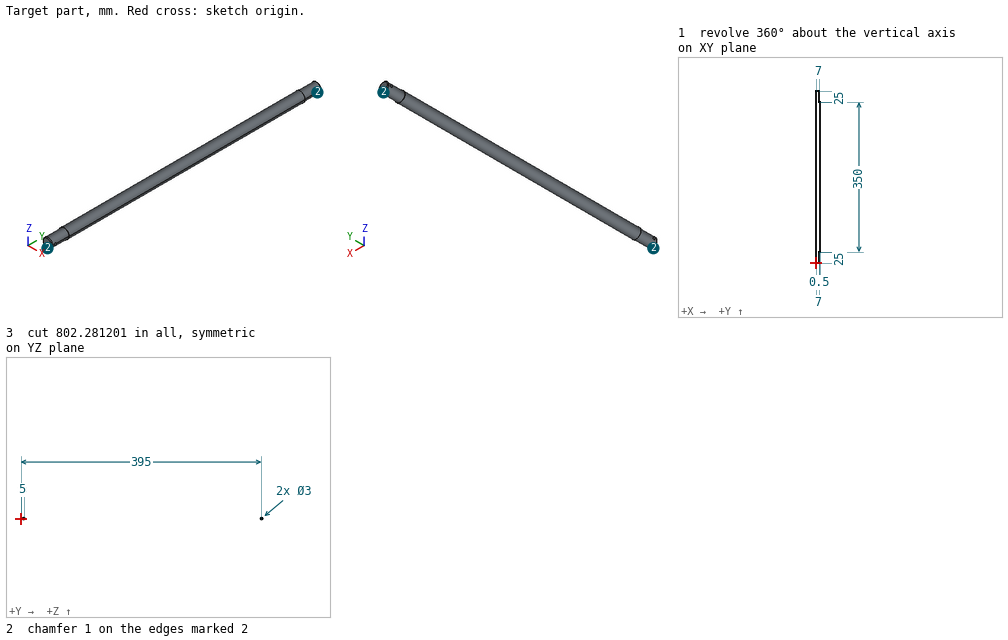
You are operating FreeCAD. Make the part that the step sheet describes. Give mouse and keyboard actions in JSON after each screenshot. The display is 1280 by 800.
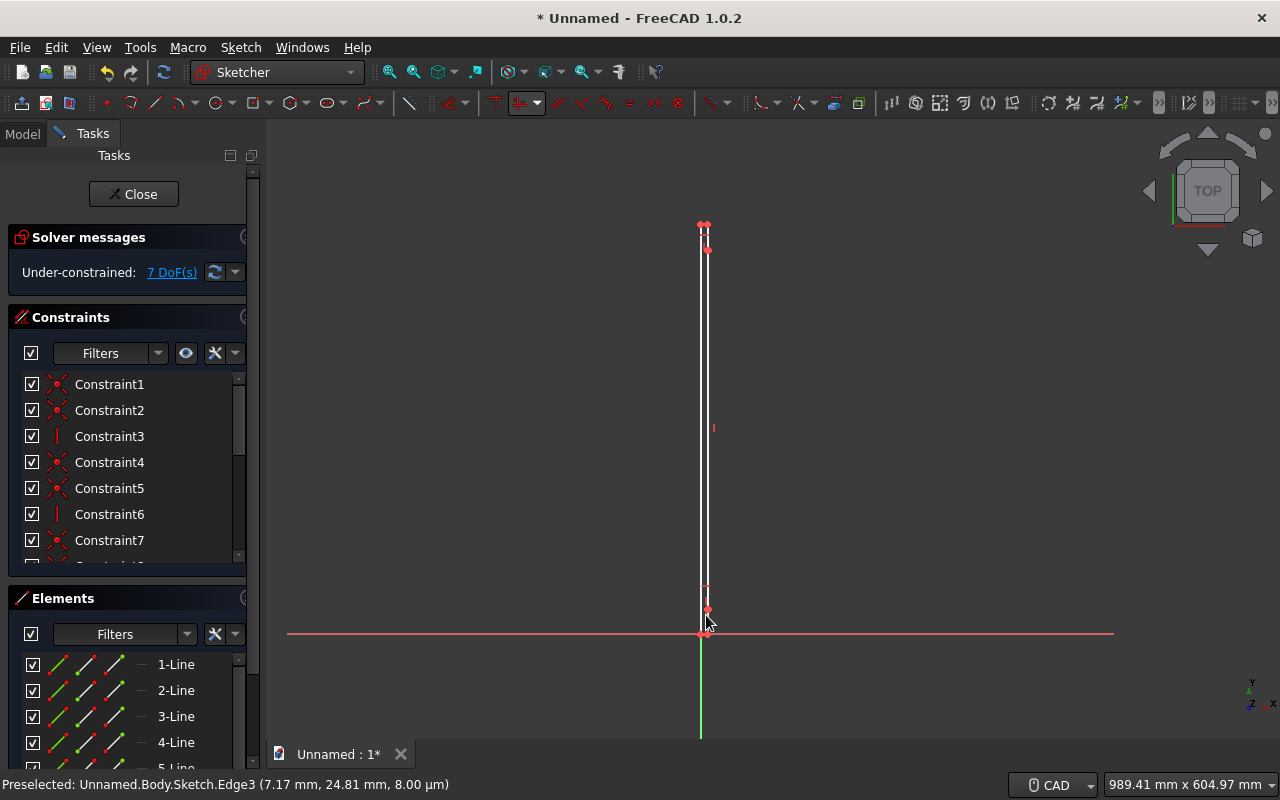
{"action": "scroll", "coordinate": [708, 250], "scroll_direction": "up", "scroll_amount": 14}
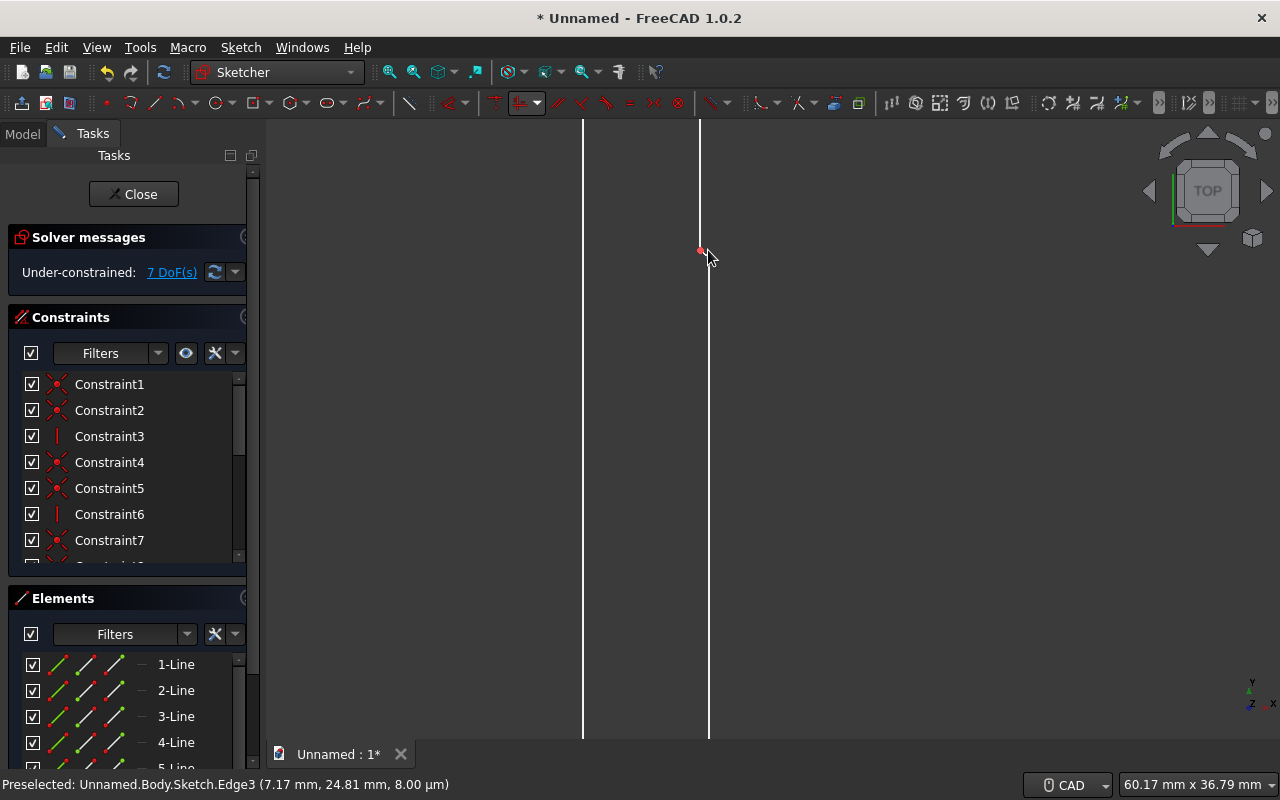
{"action": "scroll", "coordinate": [705, 254], "scroll_direction": "up", "scroll_amount": 4}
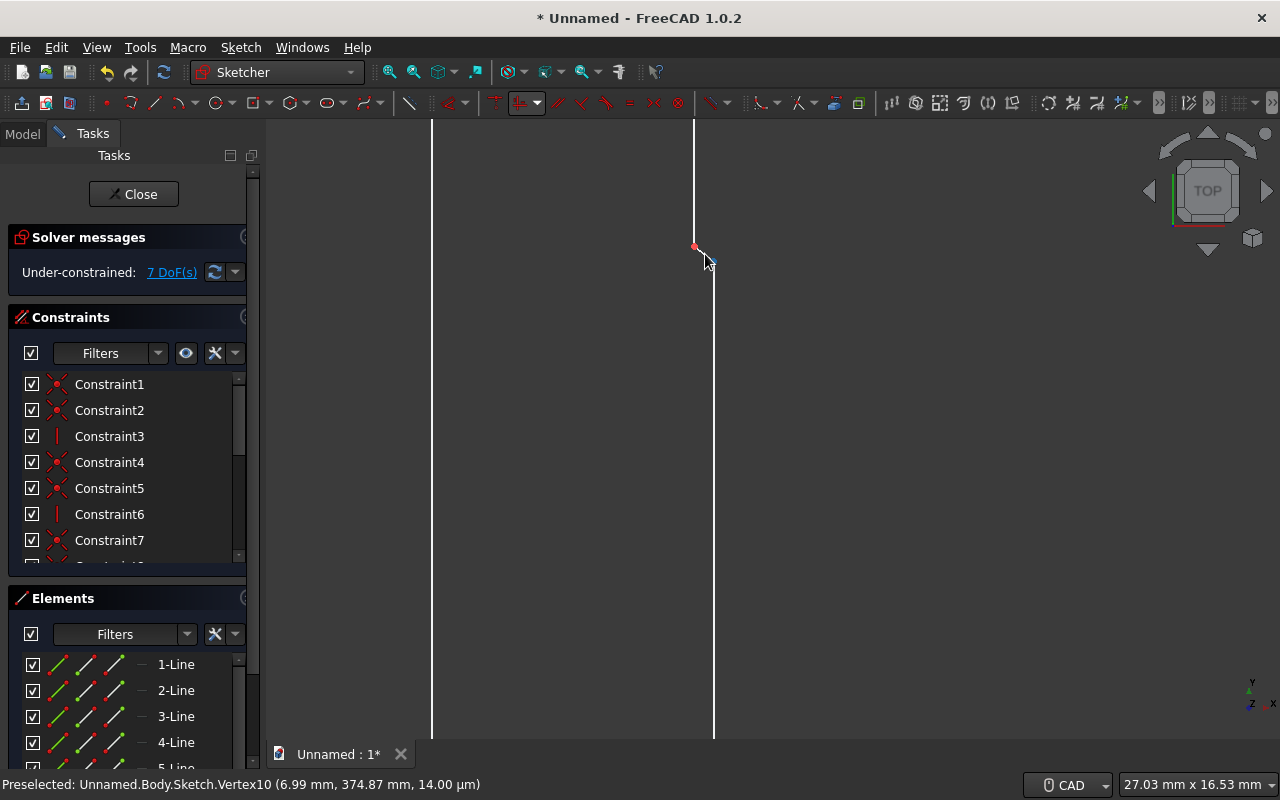
{"action": "left_click", "coordinate": [704, 254]}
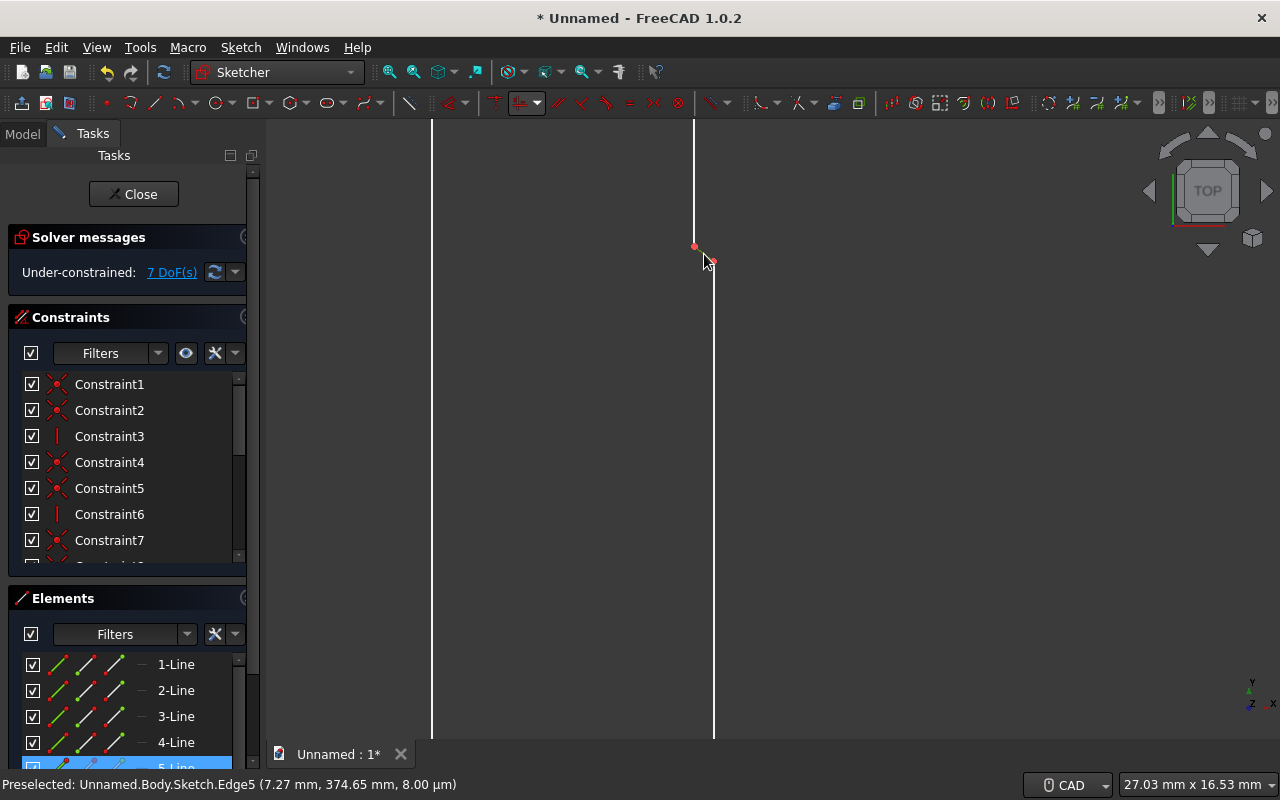
{"action": "key", "text": "h"}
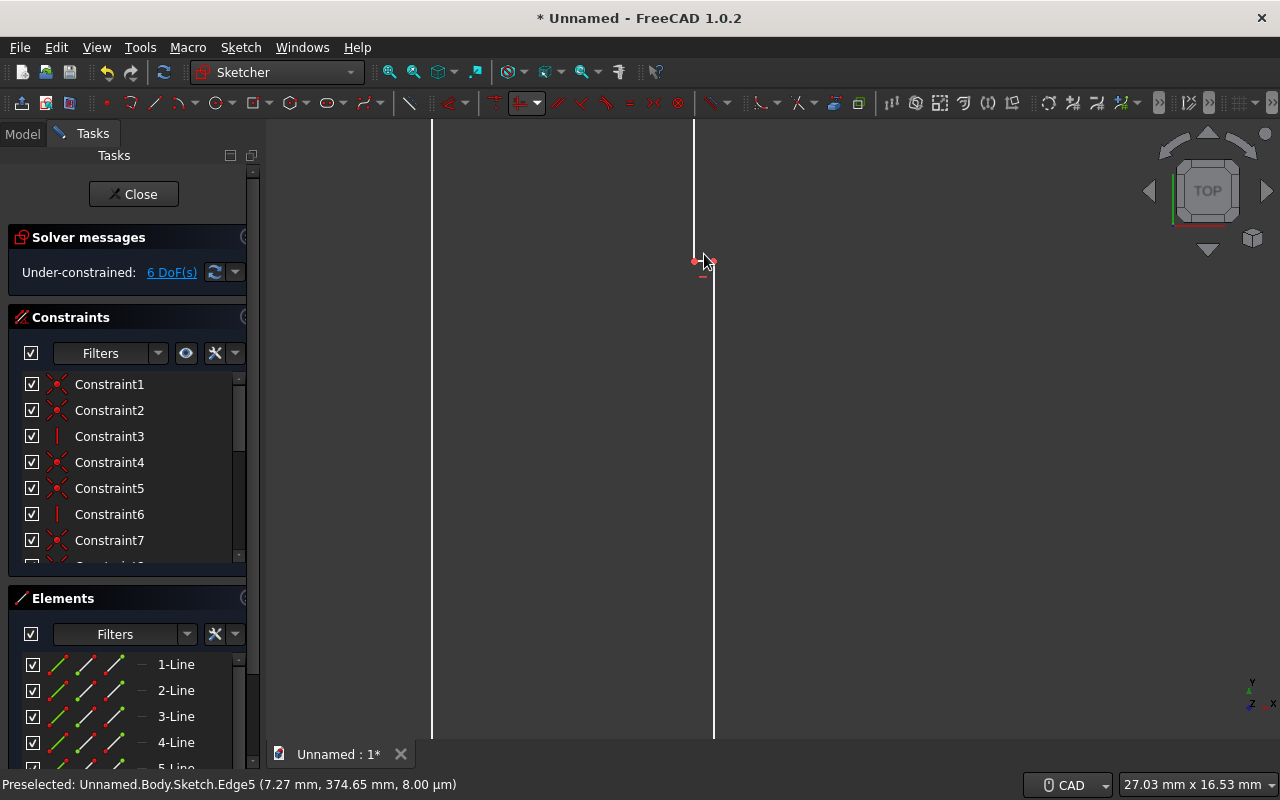
{"action": "left_click", "coordinate": [448, 104]}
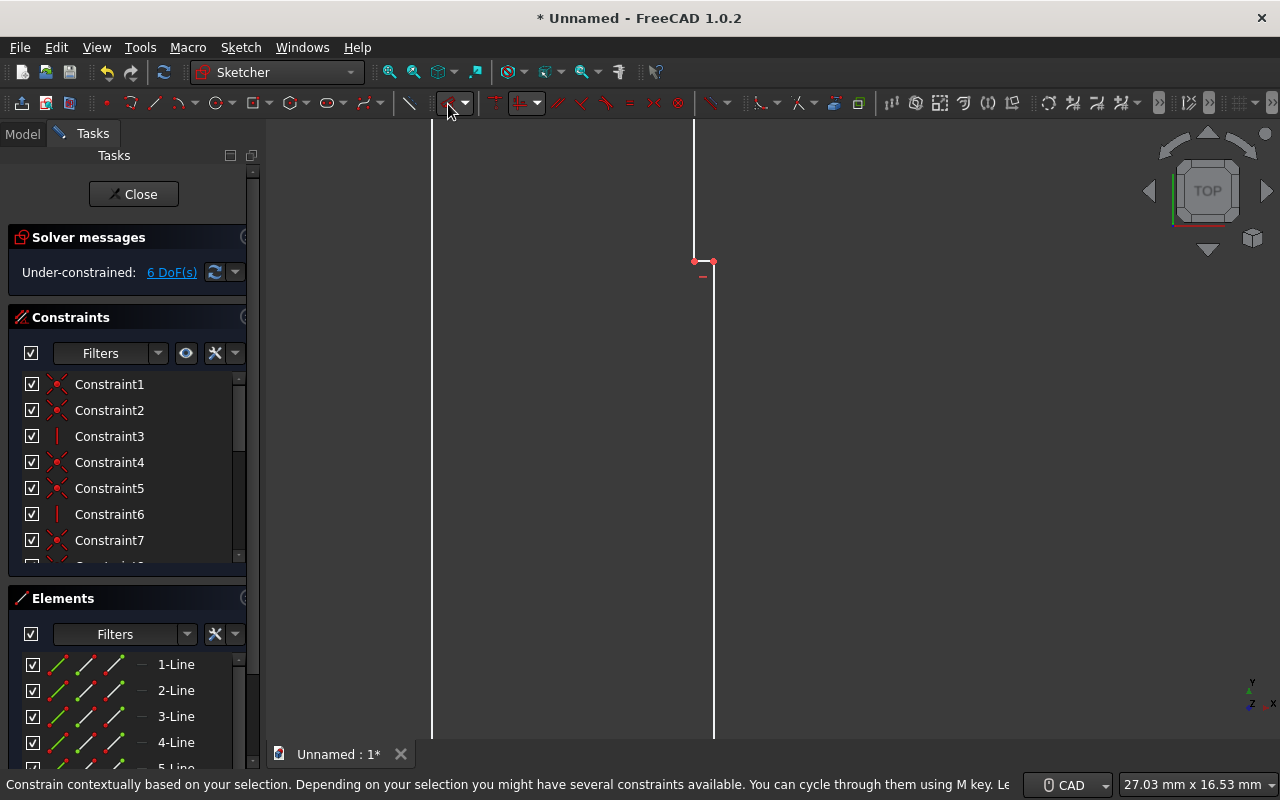
{"action": "scroll", "coordinate": [709, 209], "scroll_direction": "down", "scroll_amount": 17}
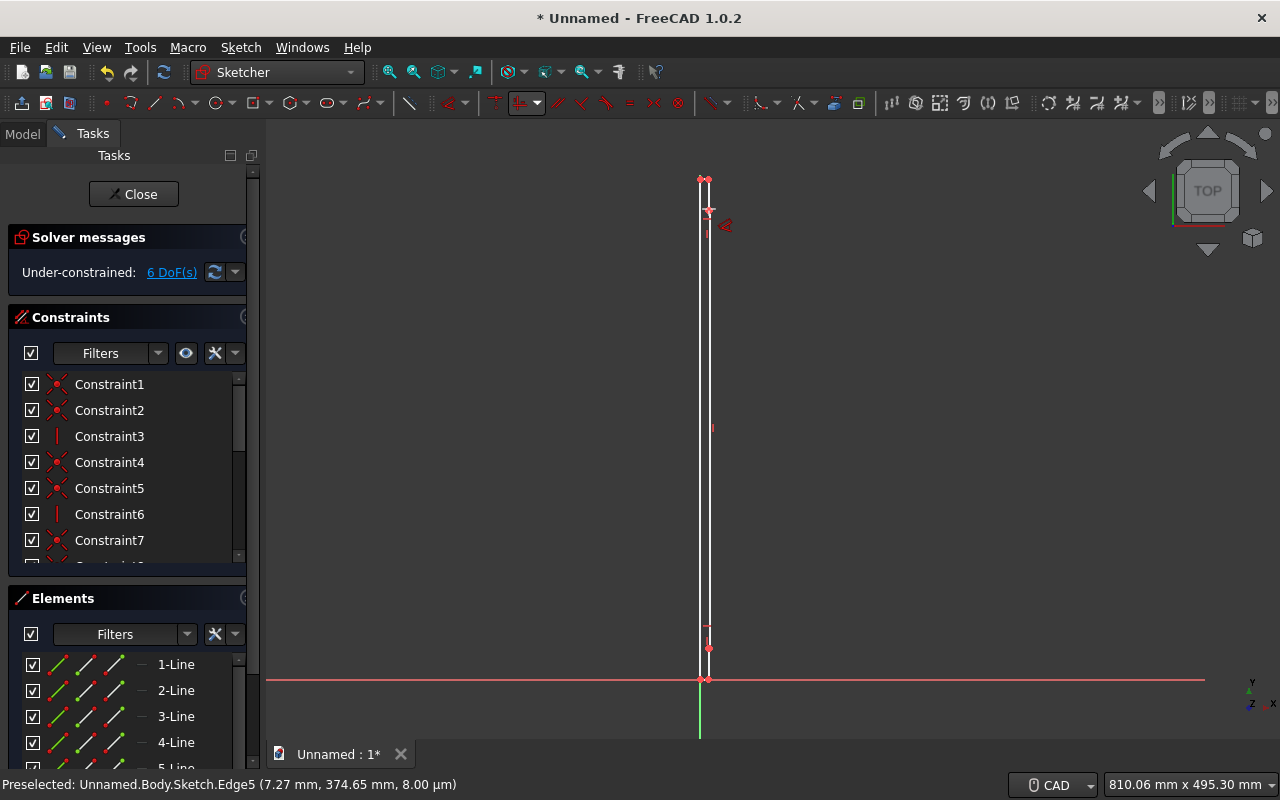
{"action": "scroll", "coordinate": [703, 680], "scroll_direction": "up", "scroll_amount": 9}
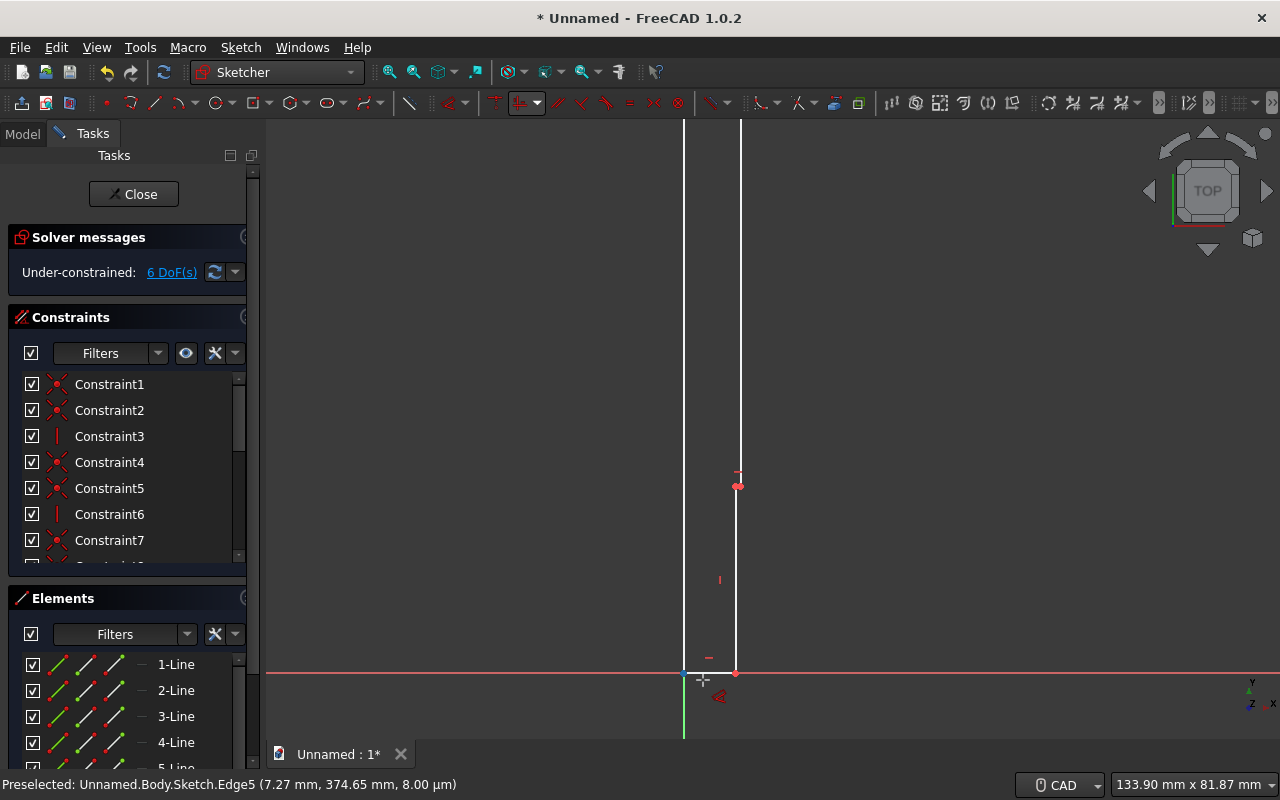
{"action": "left_click", "coordinate": [699, 673]}
{"action": "left_click", "coordinate": [710, 707]}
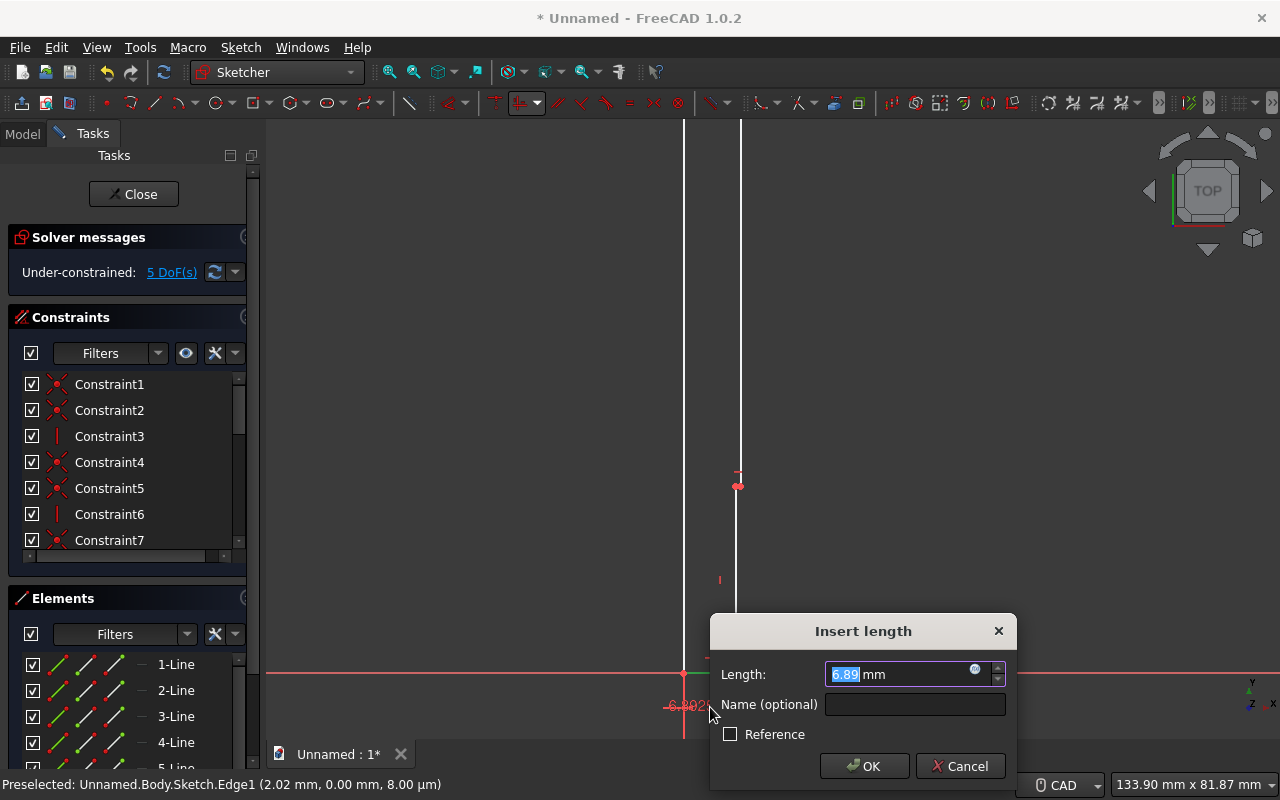
{"action": "type", "text": "7"}
{"action": "key", "text": "Return"}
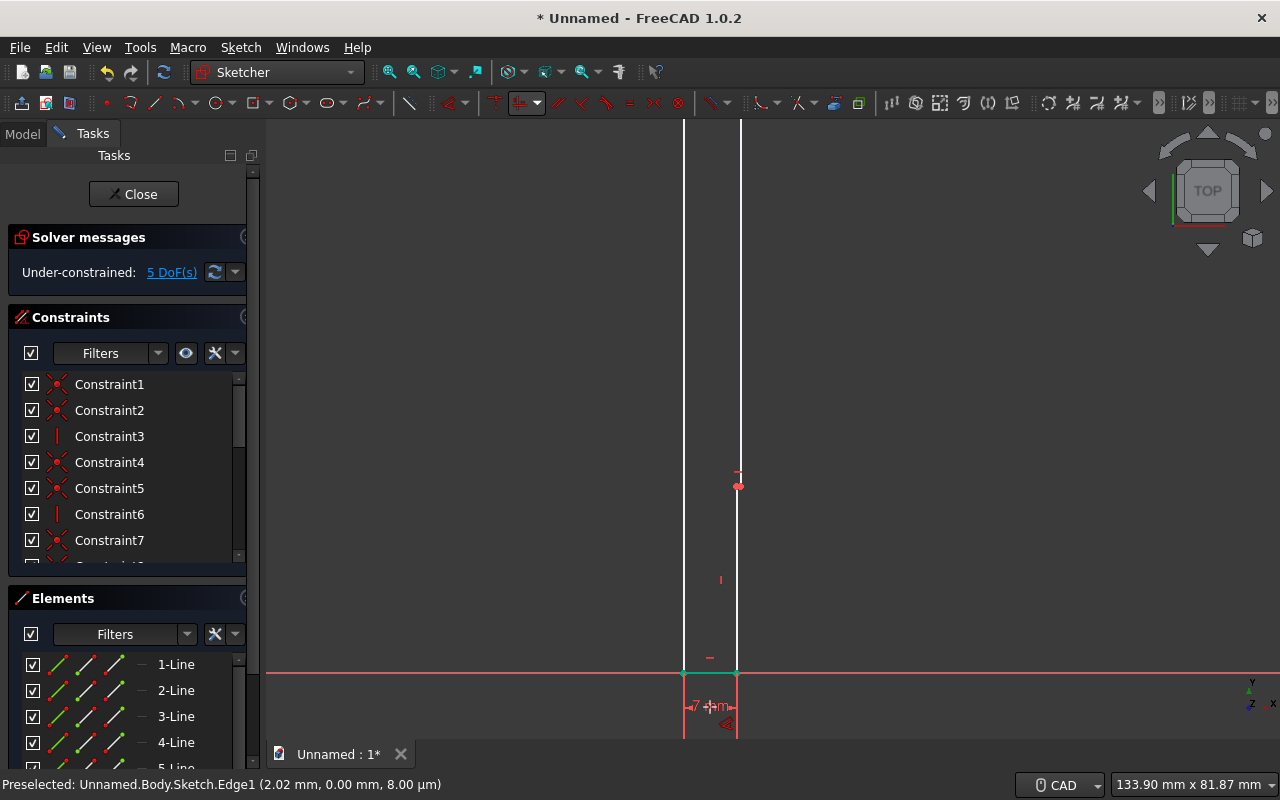
{"action": "scroll", "coordinate": [703, 628], "scroll_direction": "down", "scroll_amount": 10}